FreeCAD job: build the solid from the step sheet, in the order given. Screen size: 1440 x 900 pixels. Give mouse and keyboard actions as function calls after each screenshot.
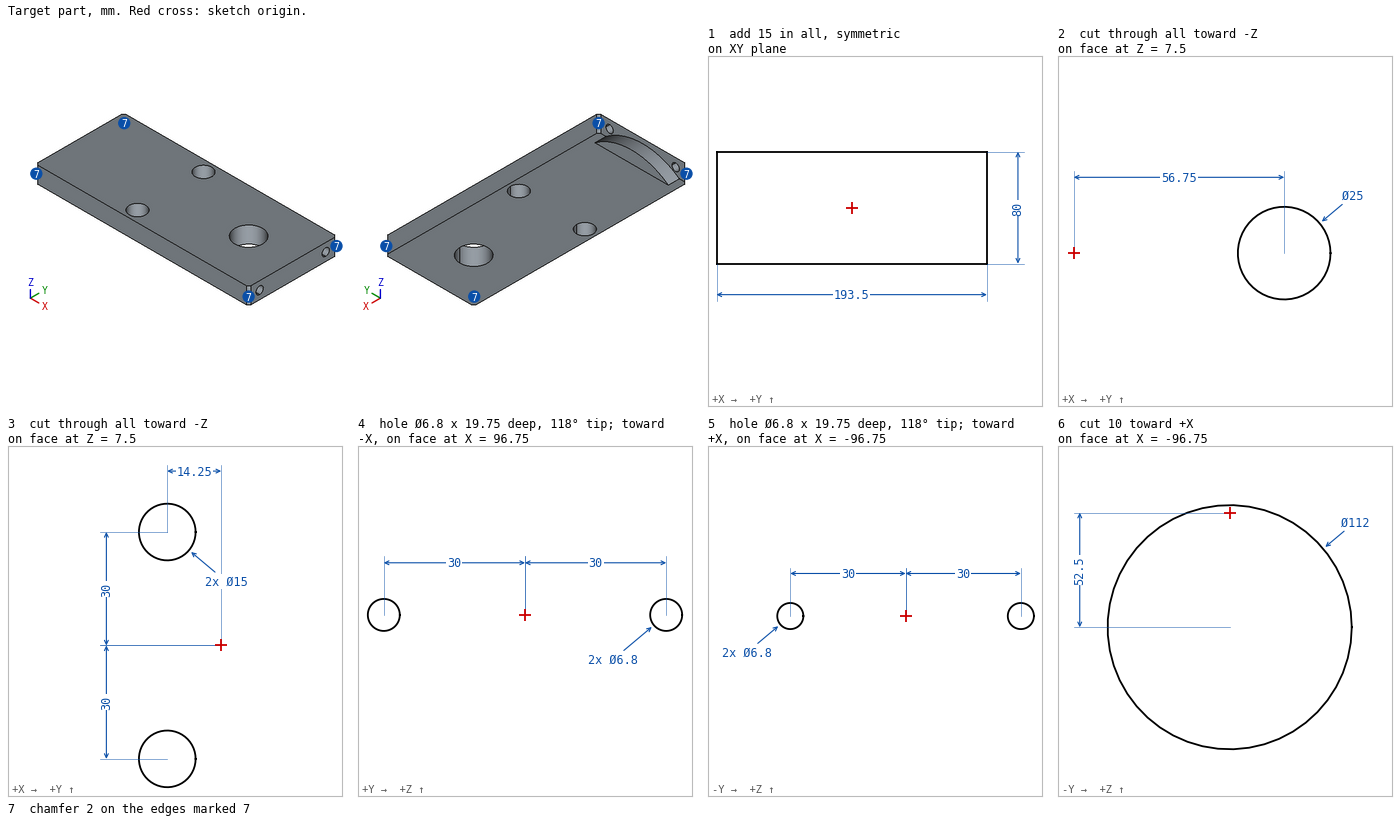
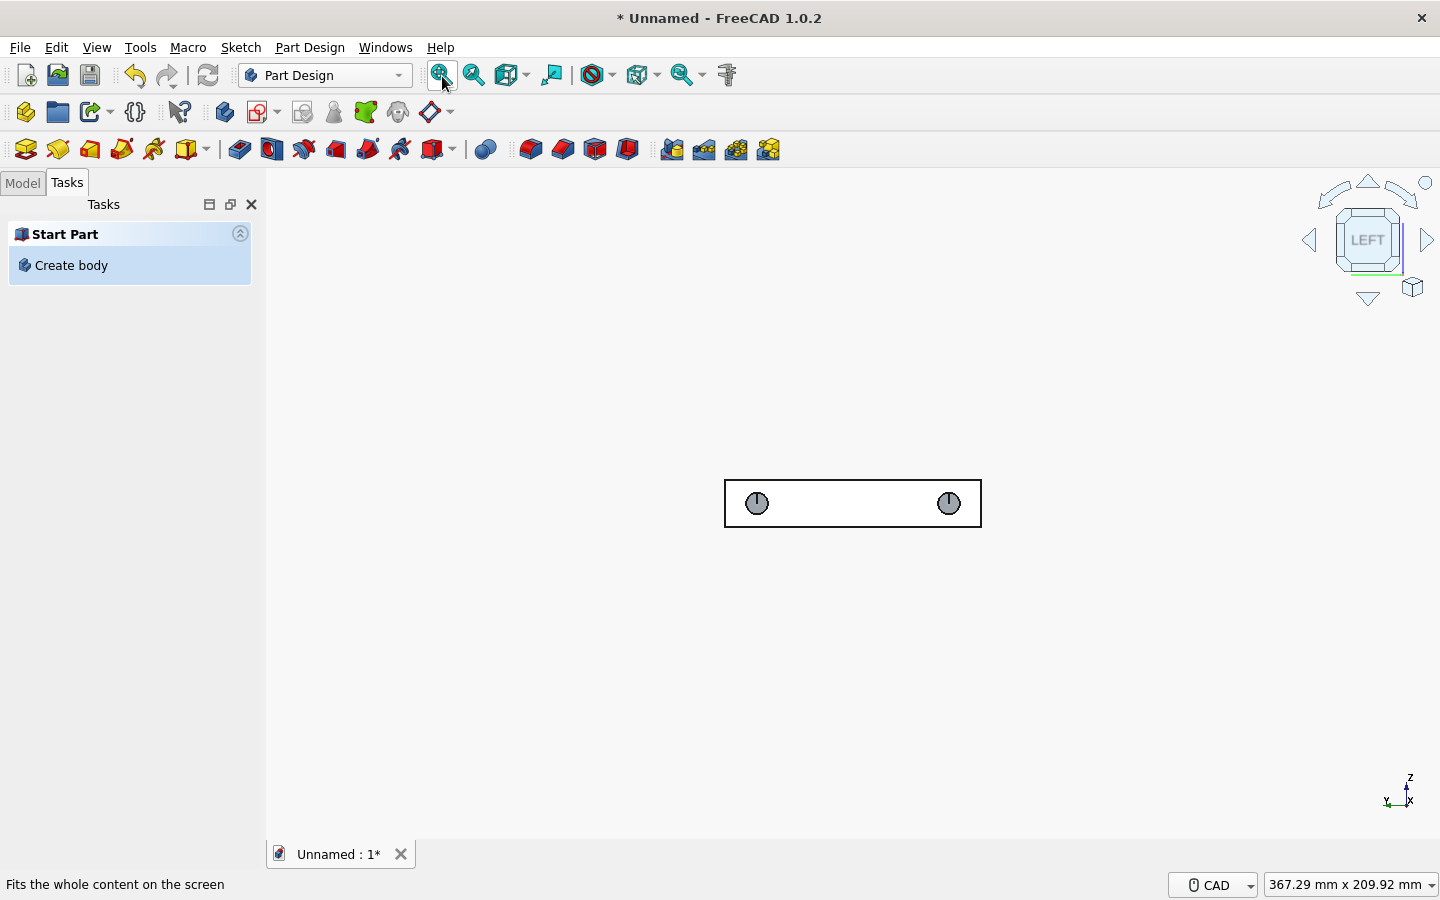
click(816, 502)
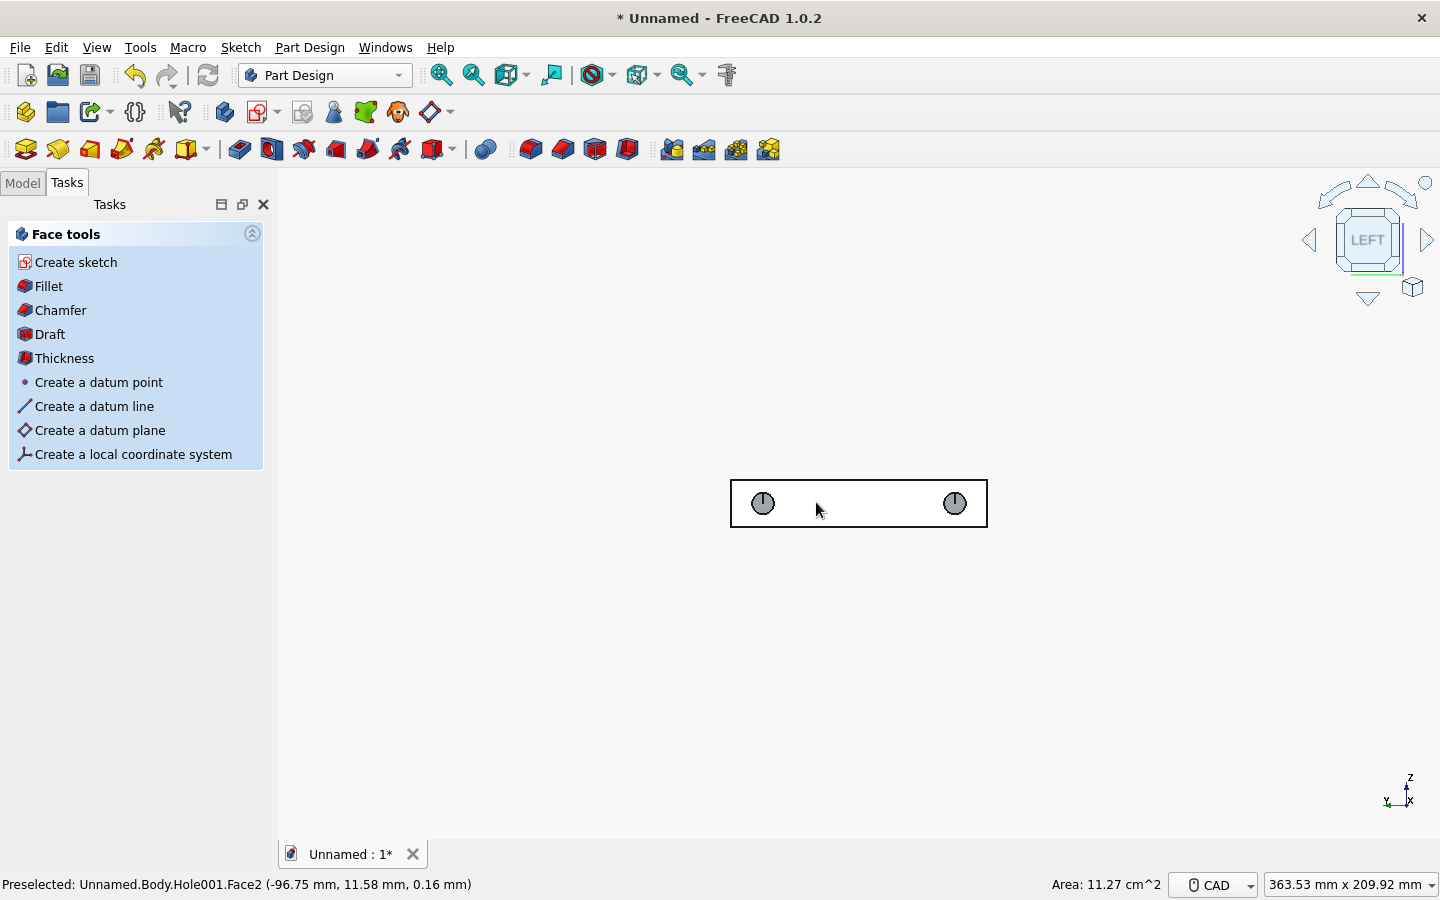
click(258, 112)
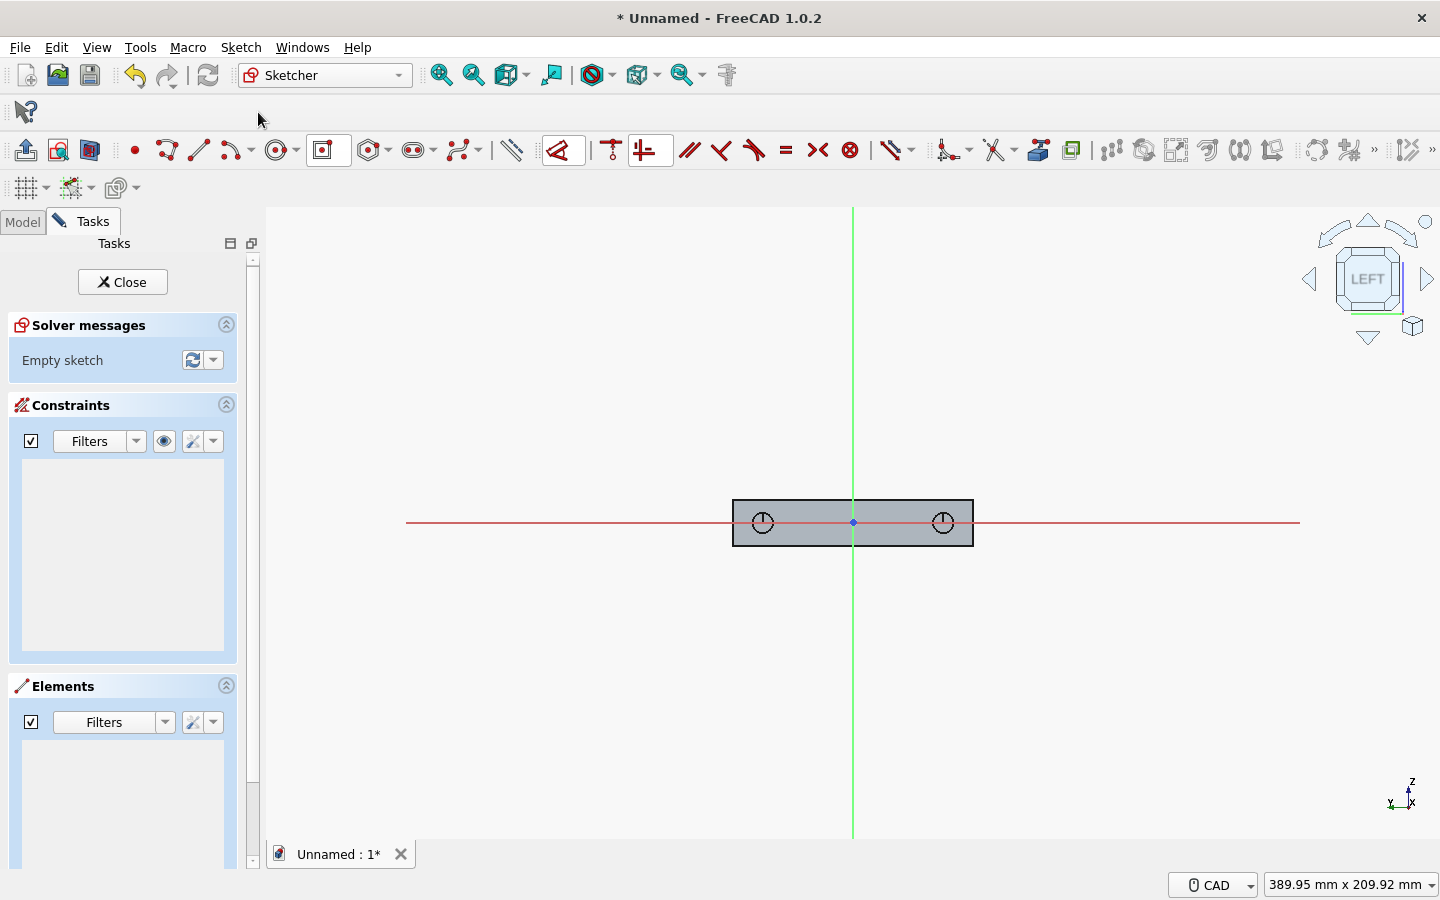
scroll(475, 235, down, 1)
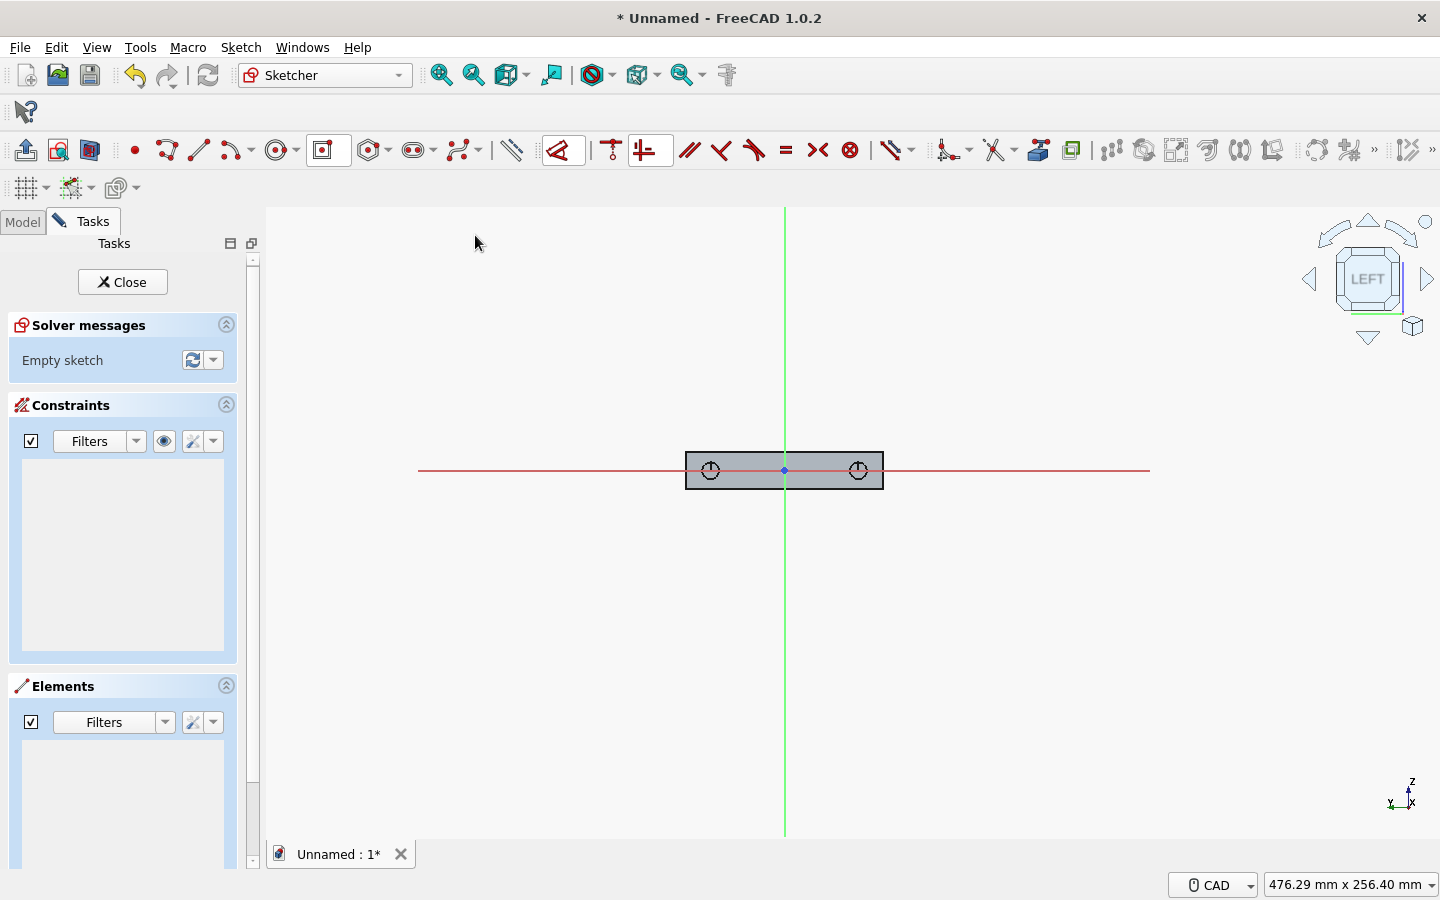
scroll(785, 757, up, 2)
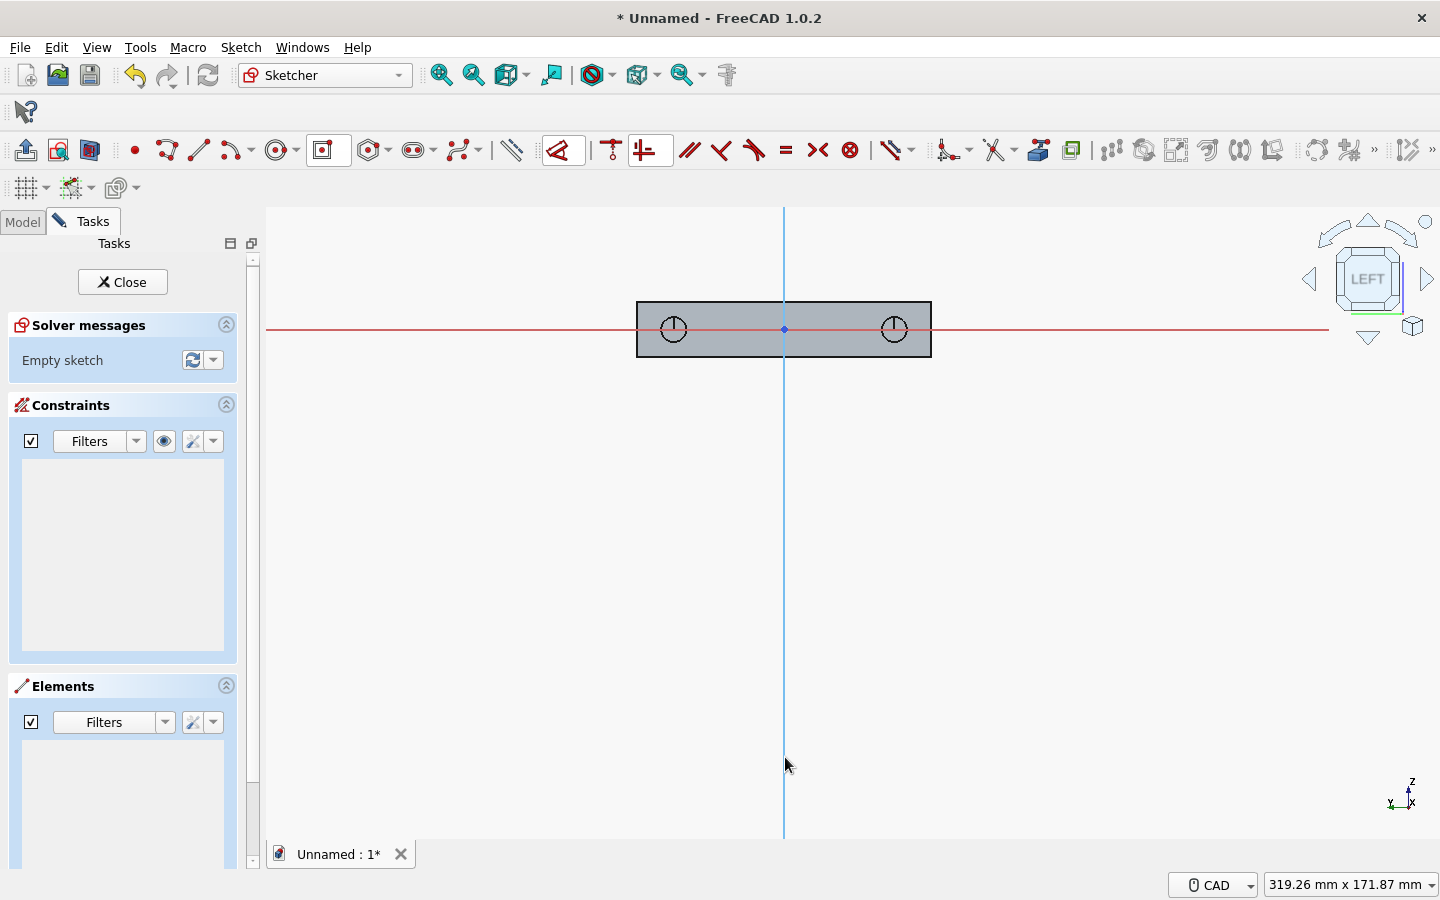
click(276, 150)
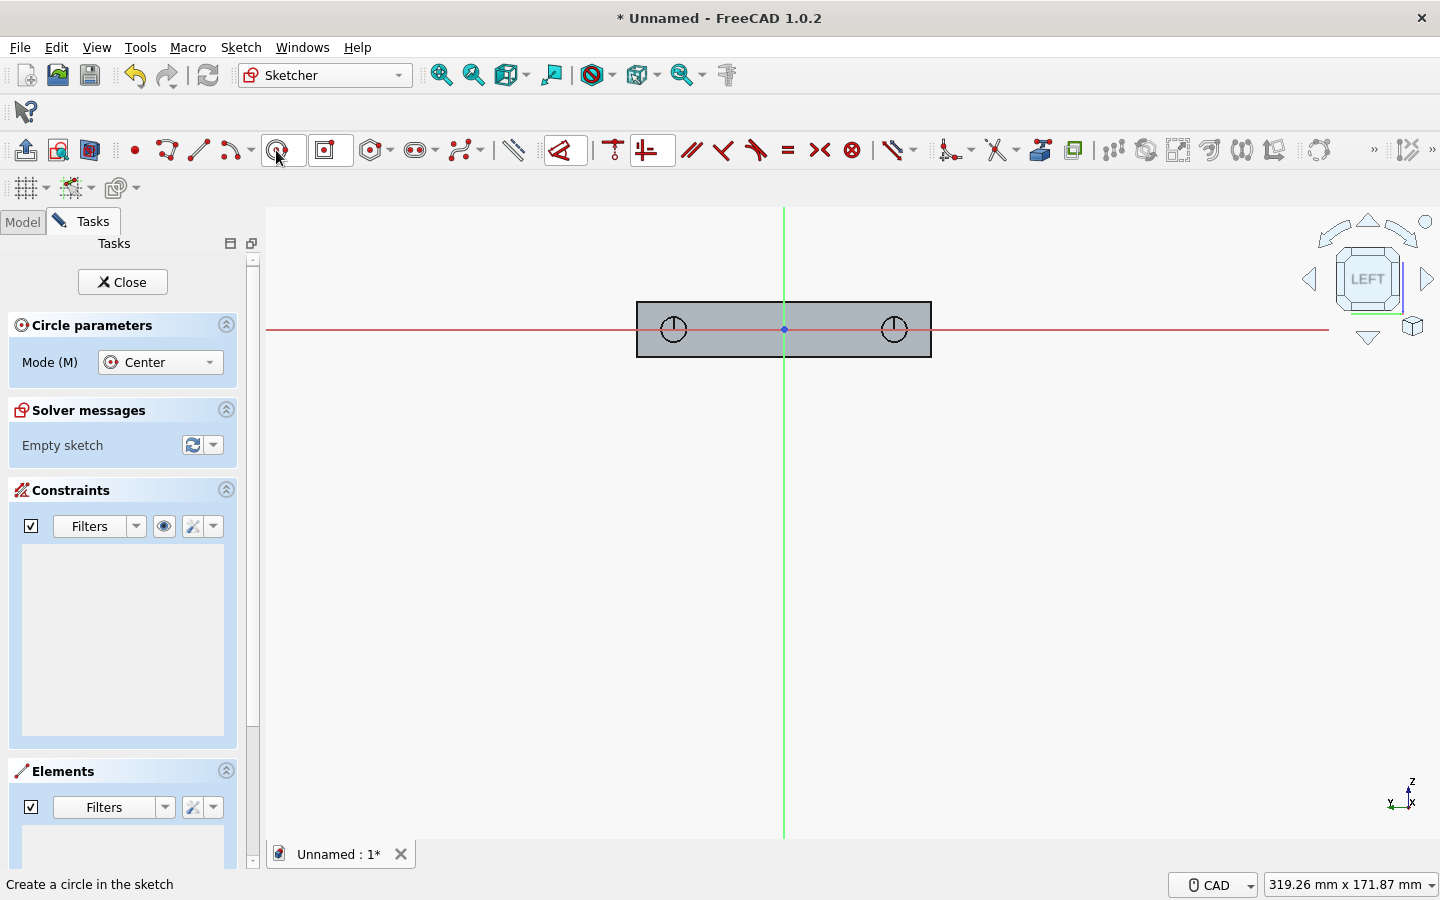
click(784, 523)
move(930, 377)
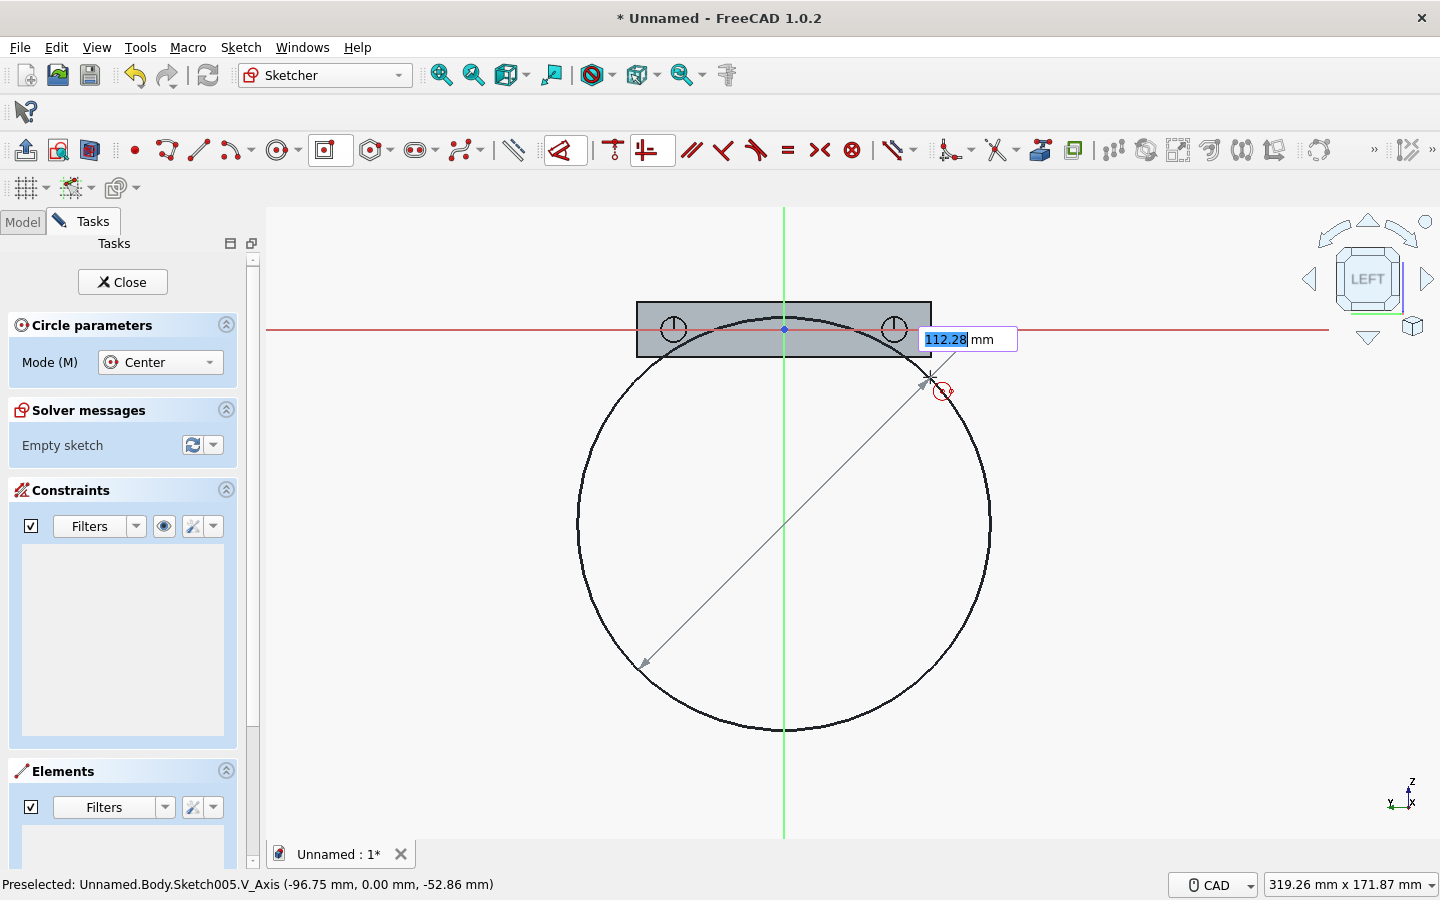
text(112)
key(Return)
key(Escape)